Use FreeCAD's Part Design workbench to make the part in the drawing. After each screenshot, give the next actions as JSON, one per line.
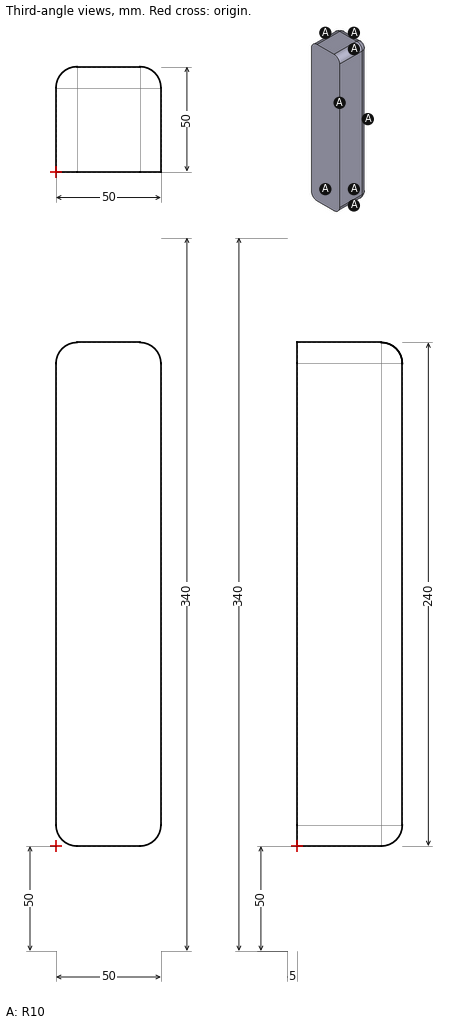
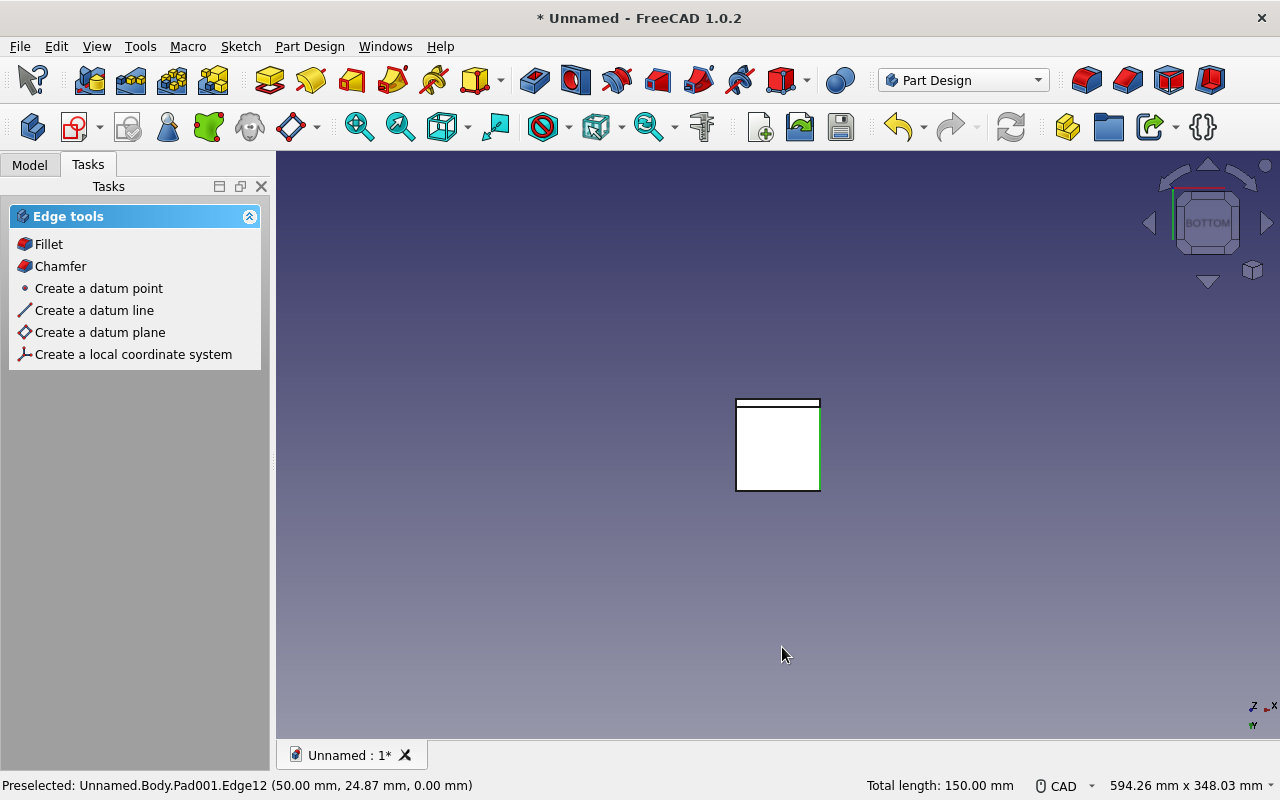
{"action": "key", "text": "v f"}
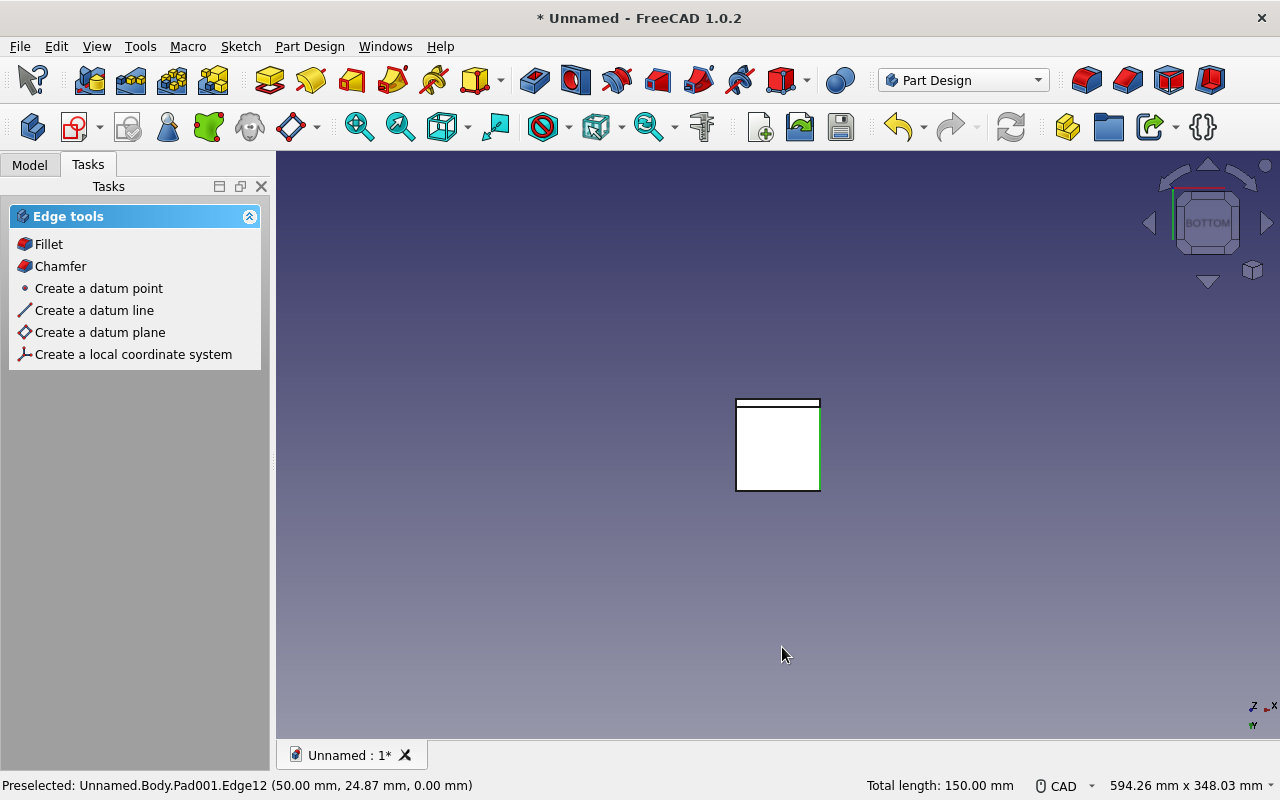
{"action": "left_click", "coordinate": [736, 448], "text": "ctrl"}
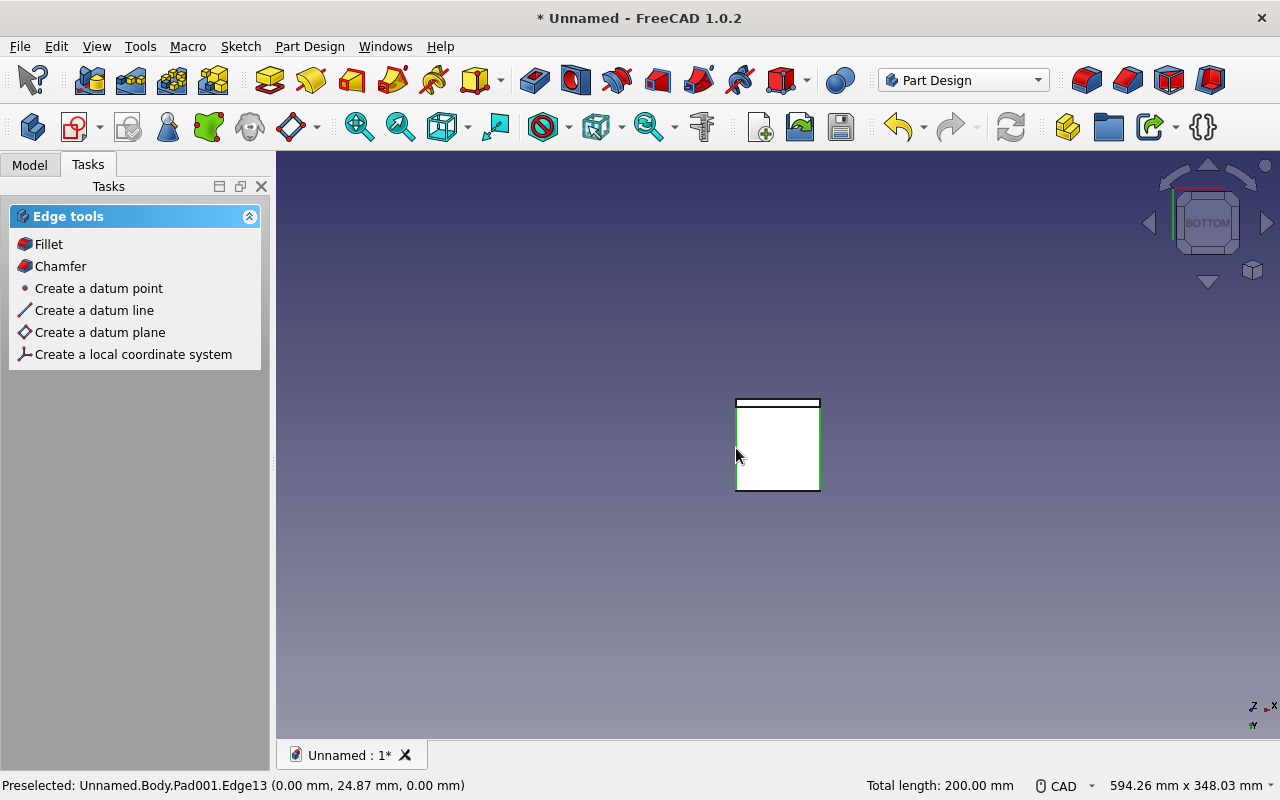
{"action": "key", "text": "4"}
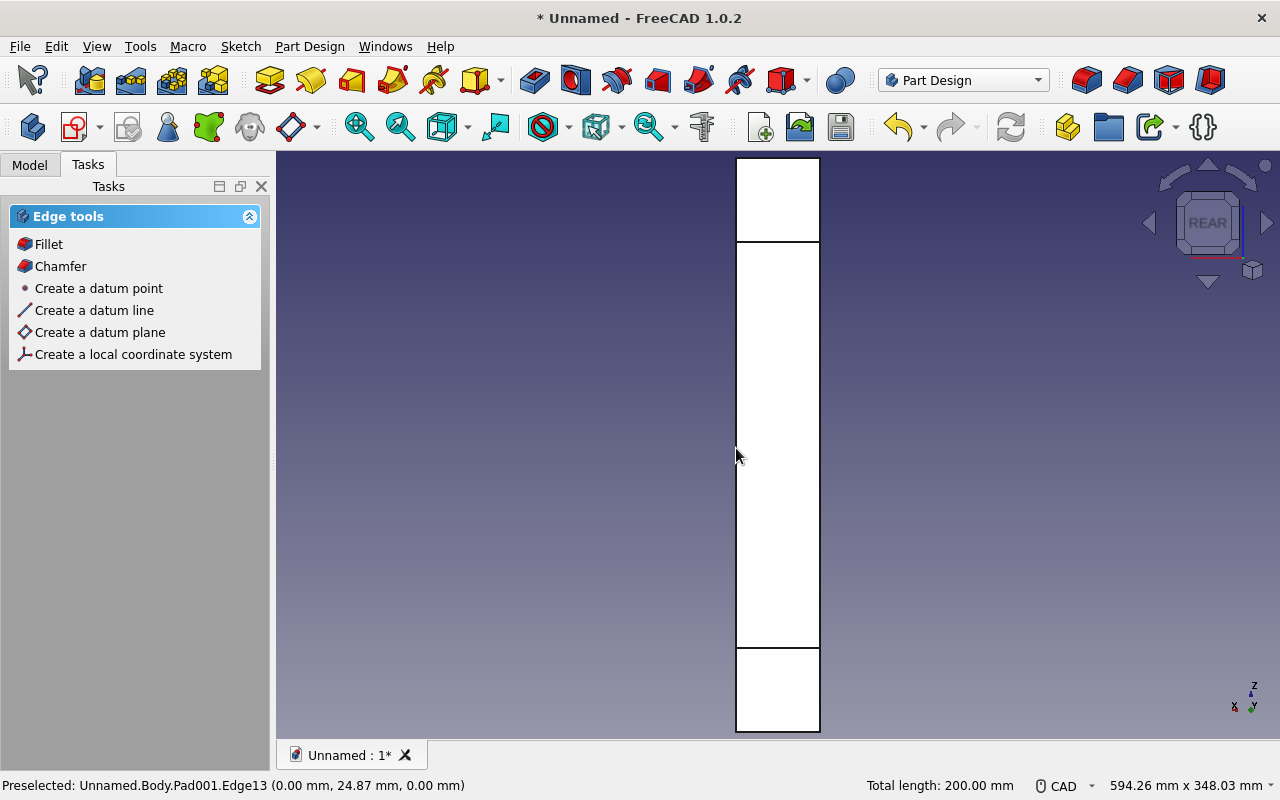
{"action": "left_click", "coordinate": [778, 328], "text": "ctrl"}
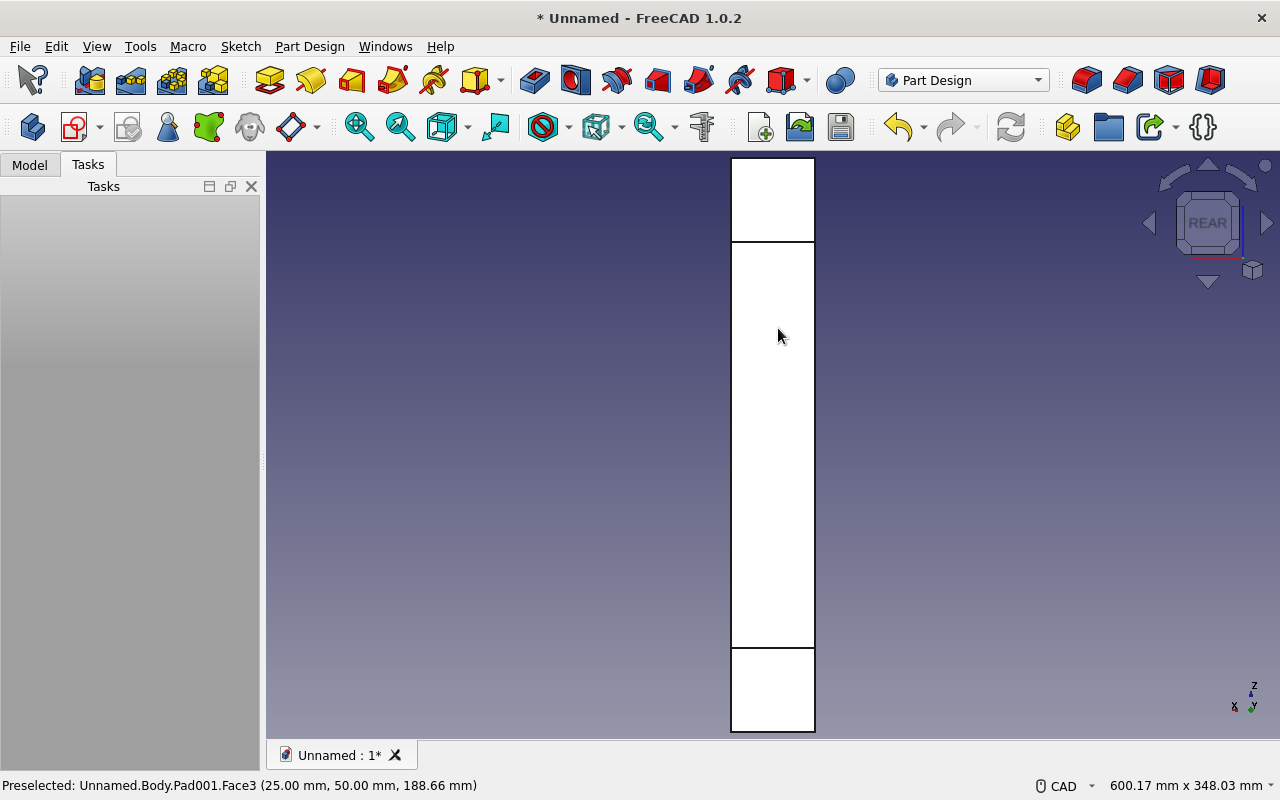
{"action": "left_click", "coordinate": [1087, 80]}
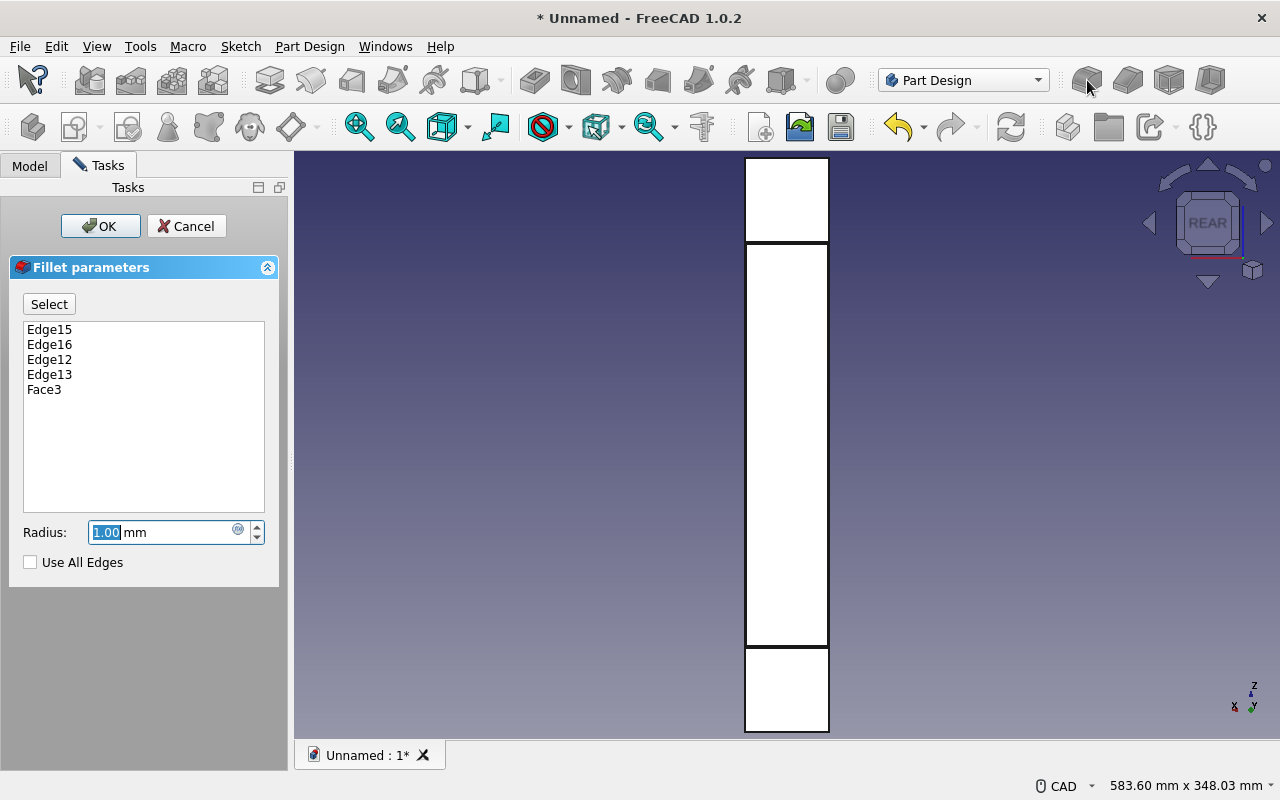
{"action": "type", "text": "10"}
{"action": "key", "text": "Tab"}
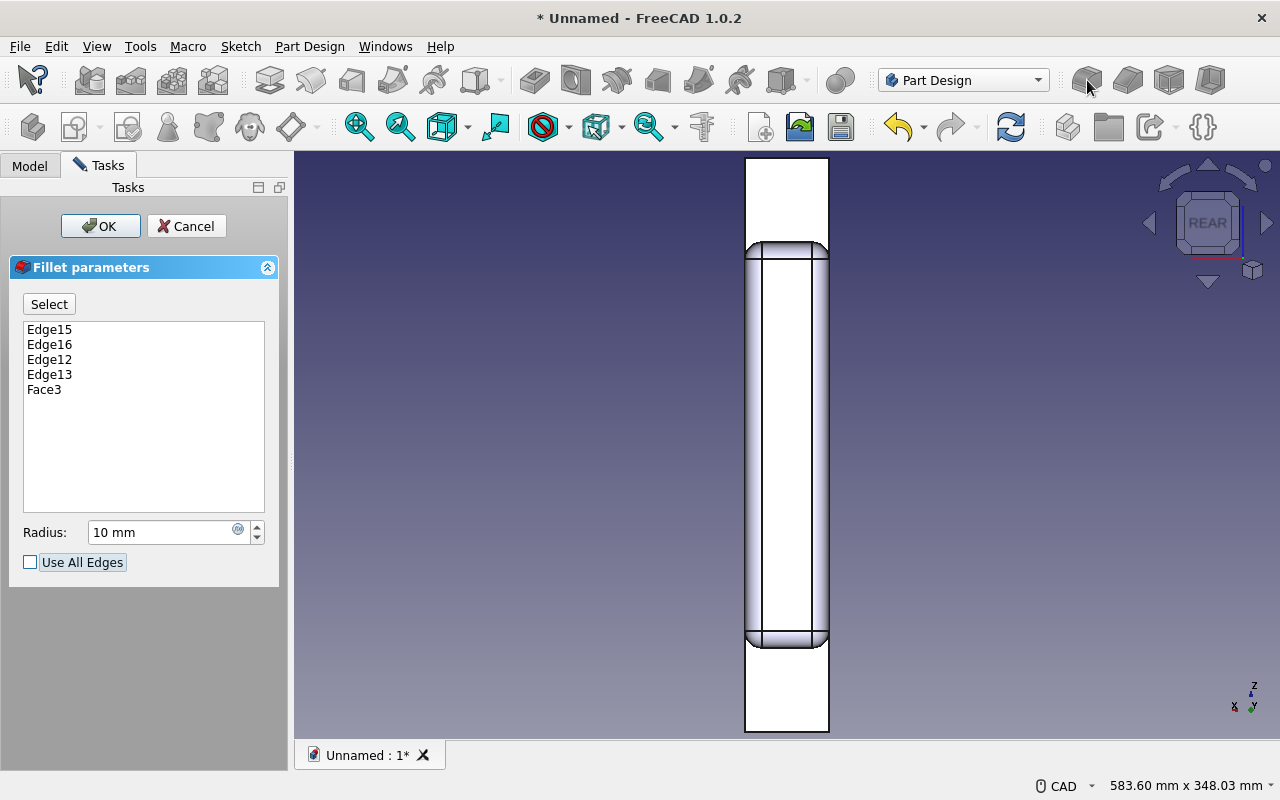
{"action": "left_click", "coordinate": [101, 226]}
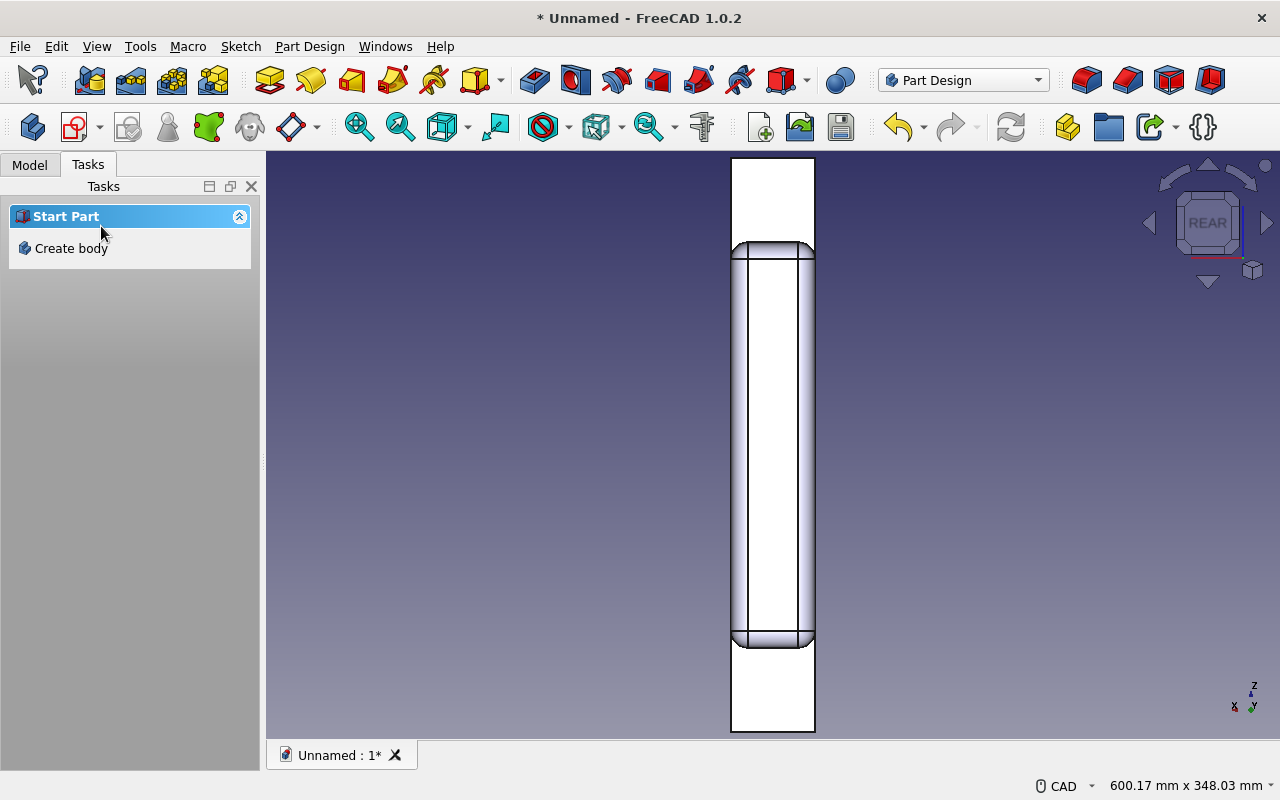
{"action": "left_click", "coordinate": [74, 128]}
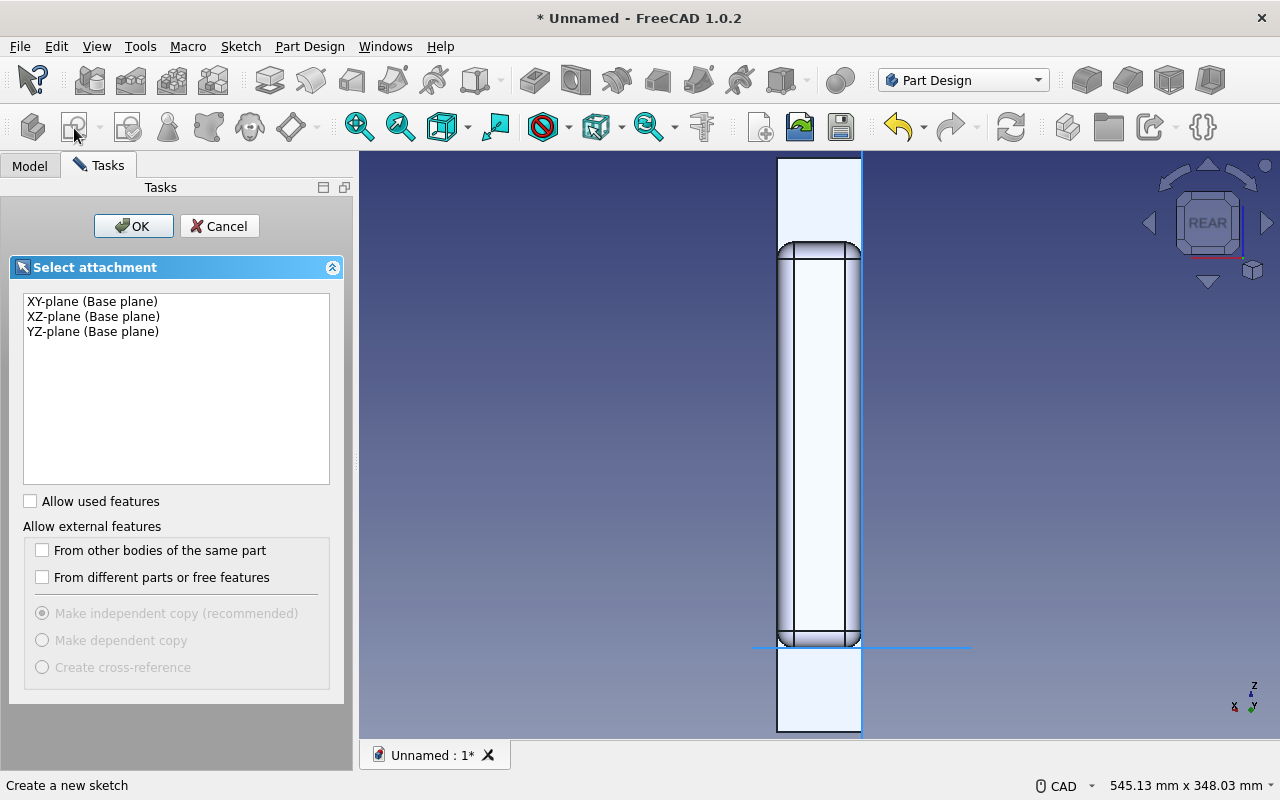
{"action": "left_click", "coordinate": [84, 332]}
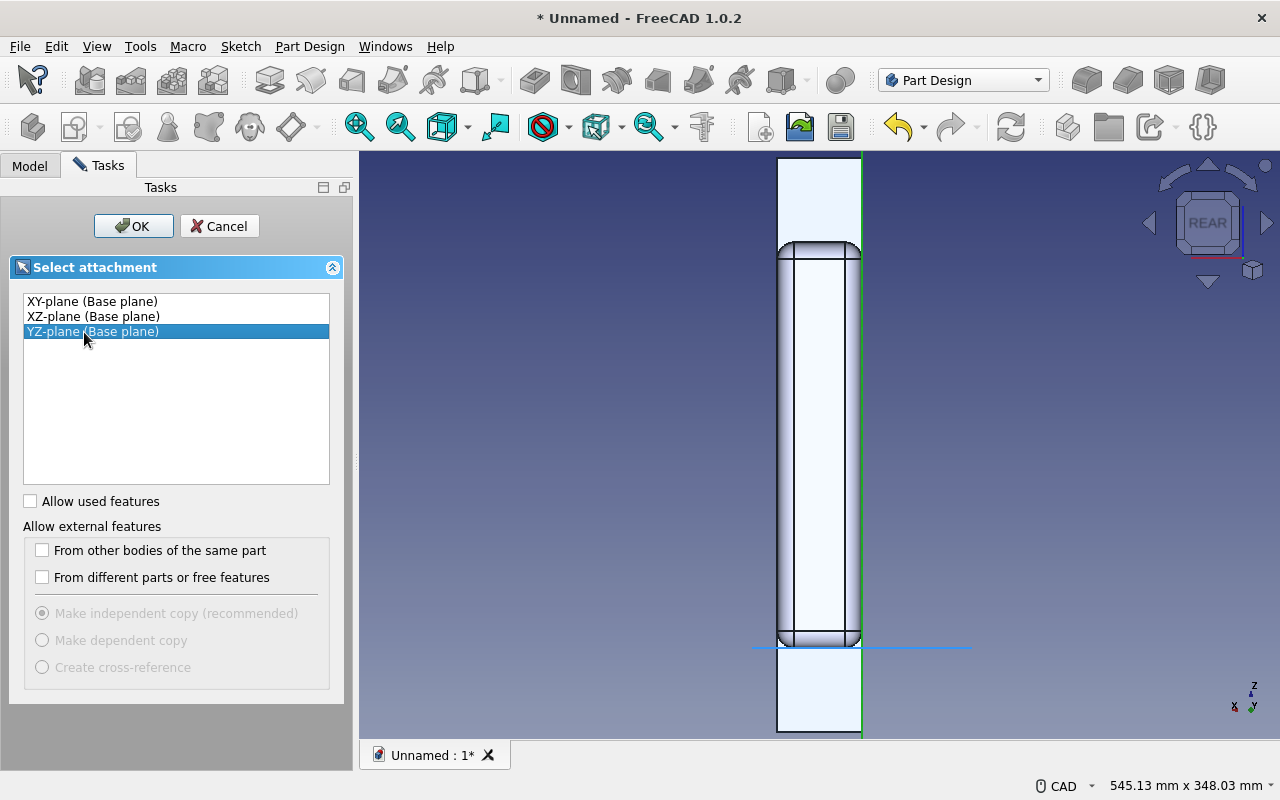
{"action": "left_click", "coordinate": [134, 226]}